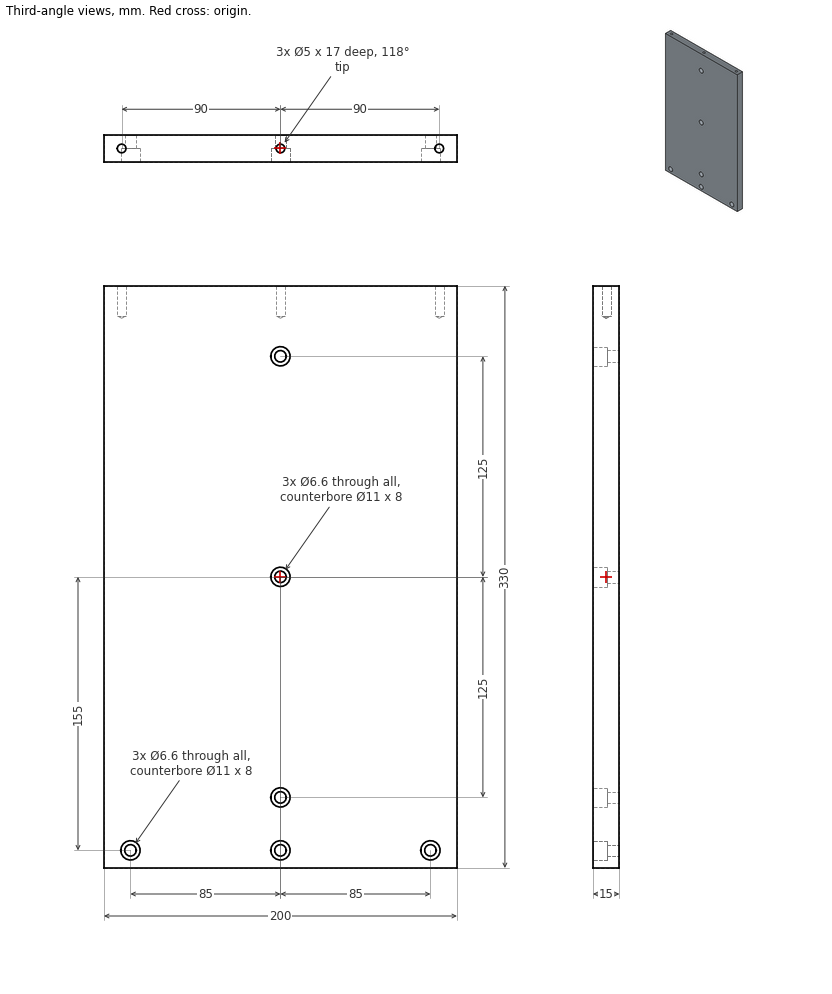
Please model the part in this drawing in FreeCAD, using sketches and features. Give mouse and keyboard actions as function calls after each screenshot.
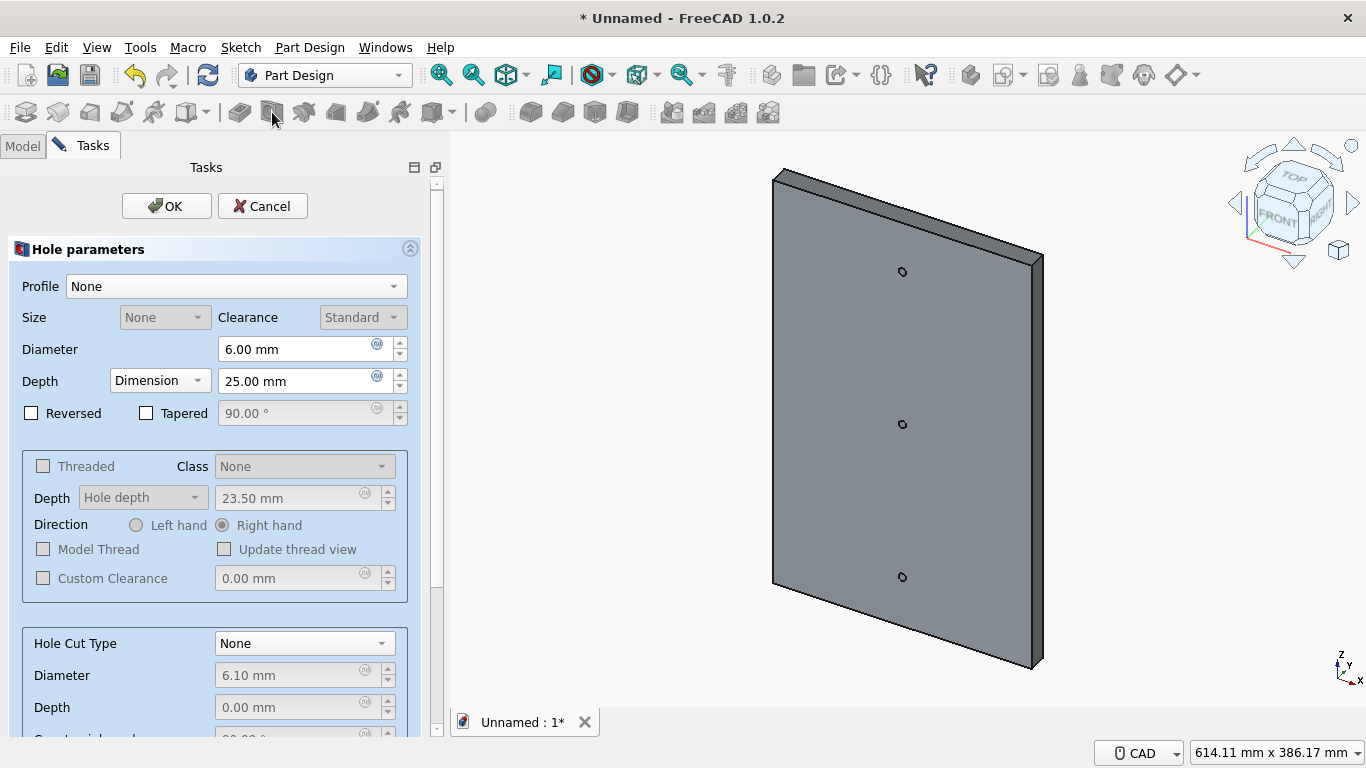
triple_click(305, 349)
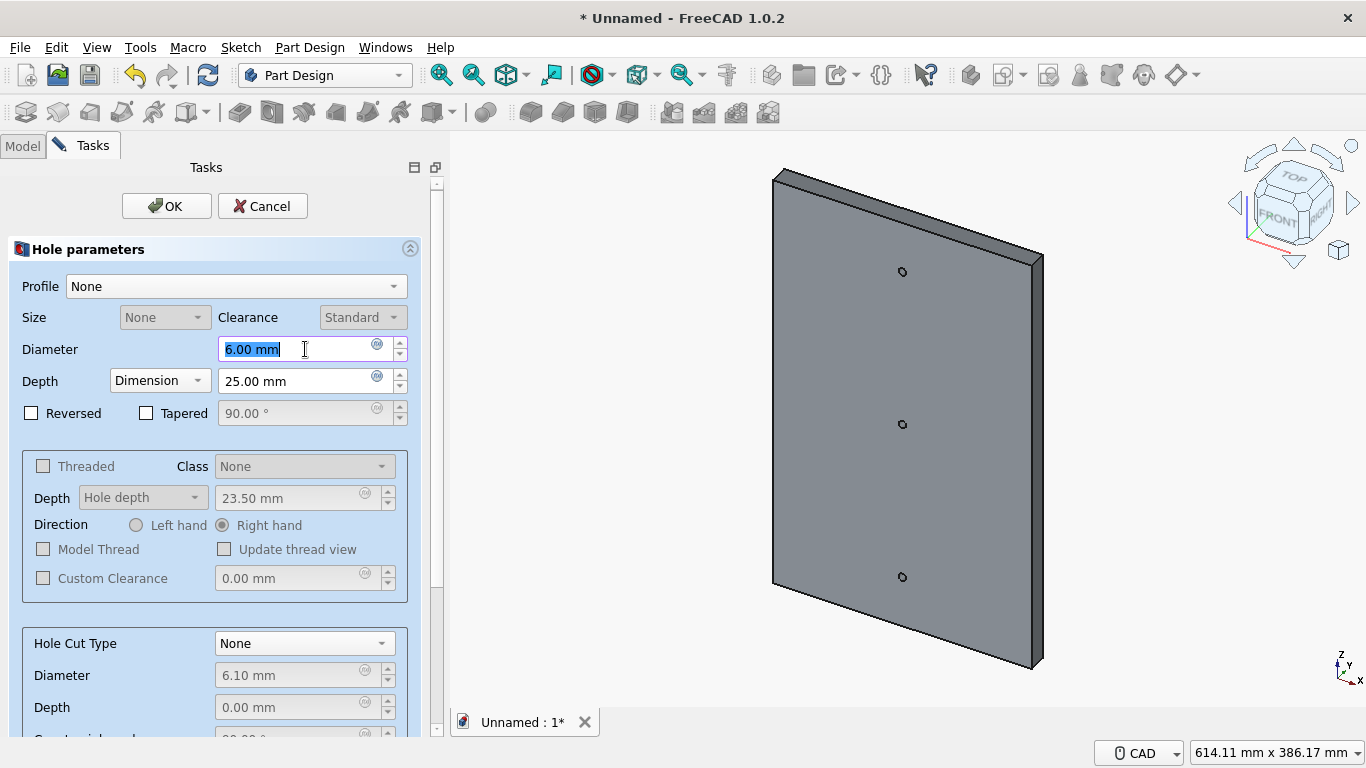
text(6.6)
key(Tab)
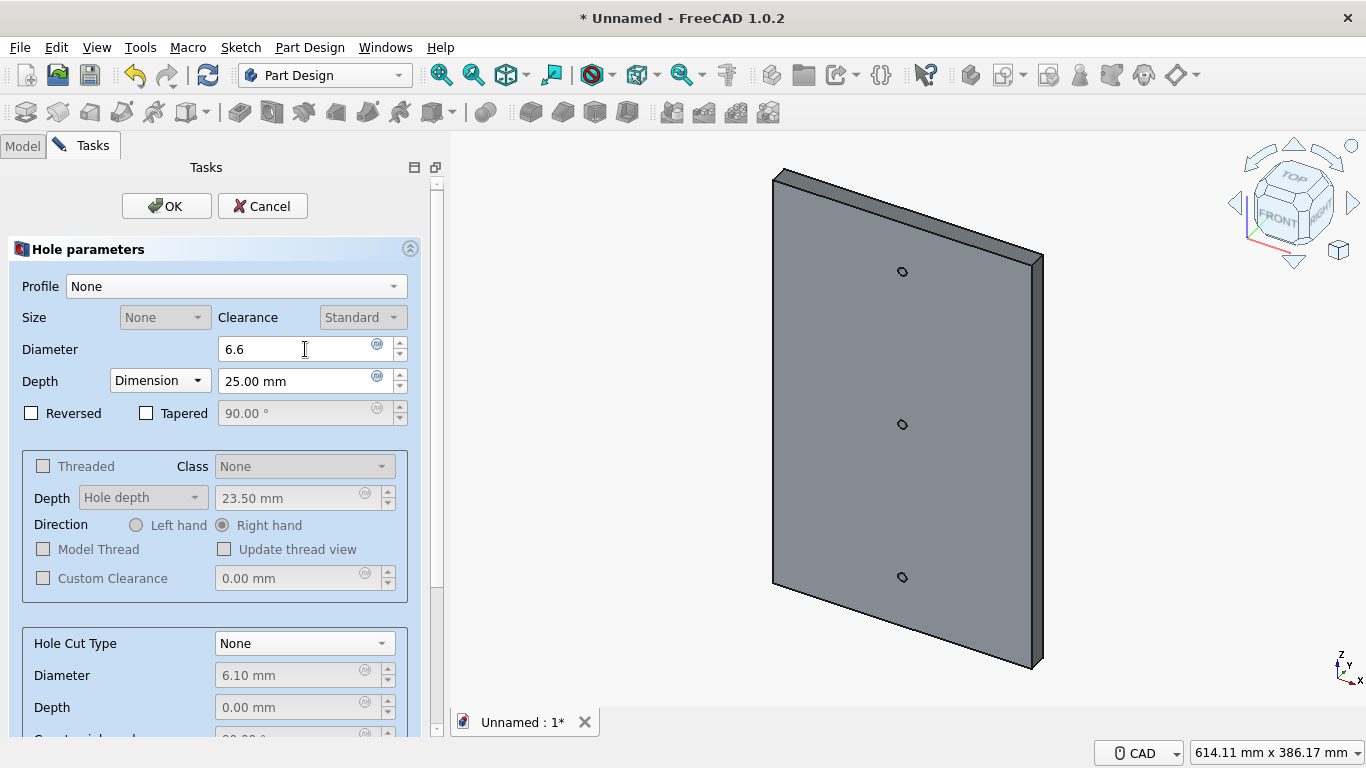
click(161, 380)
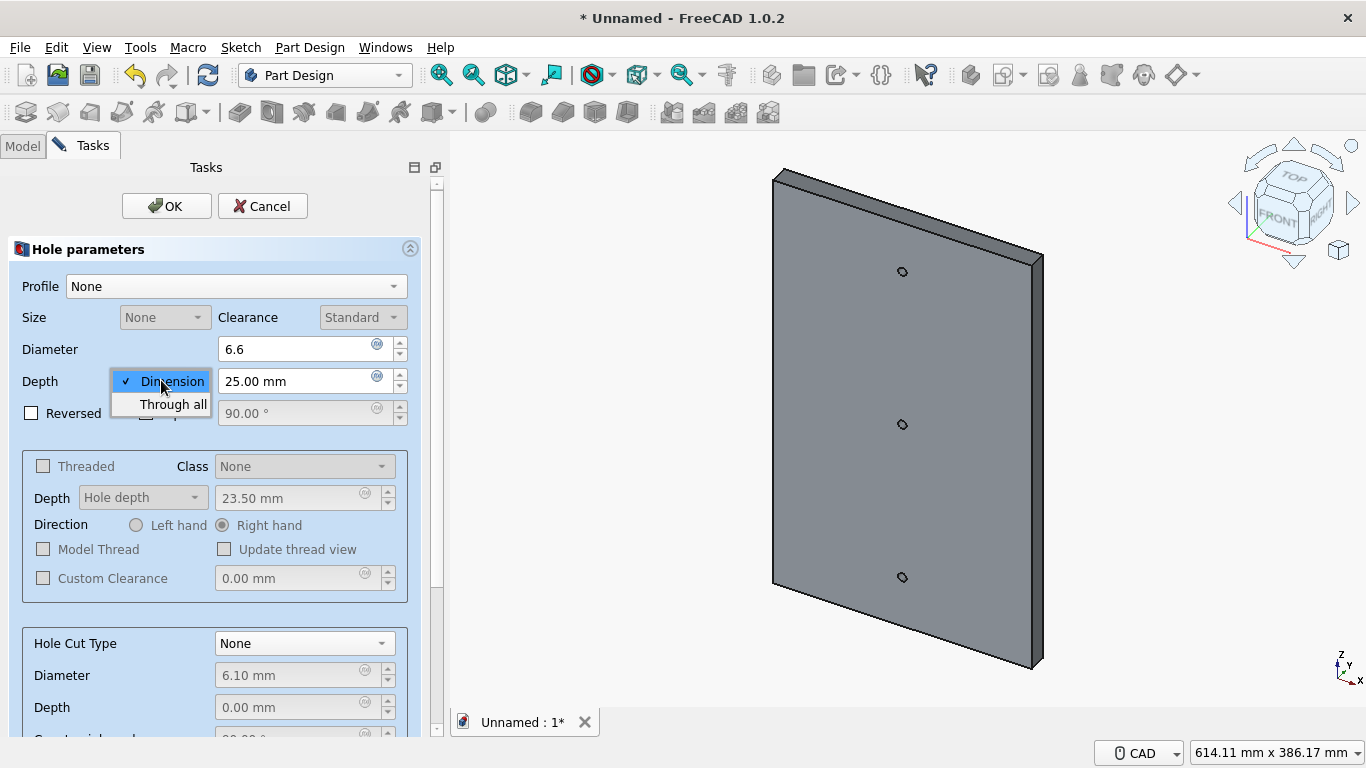
click(160, 404)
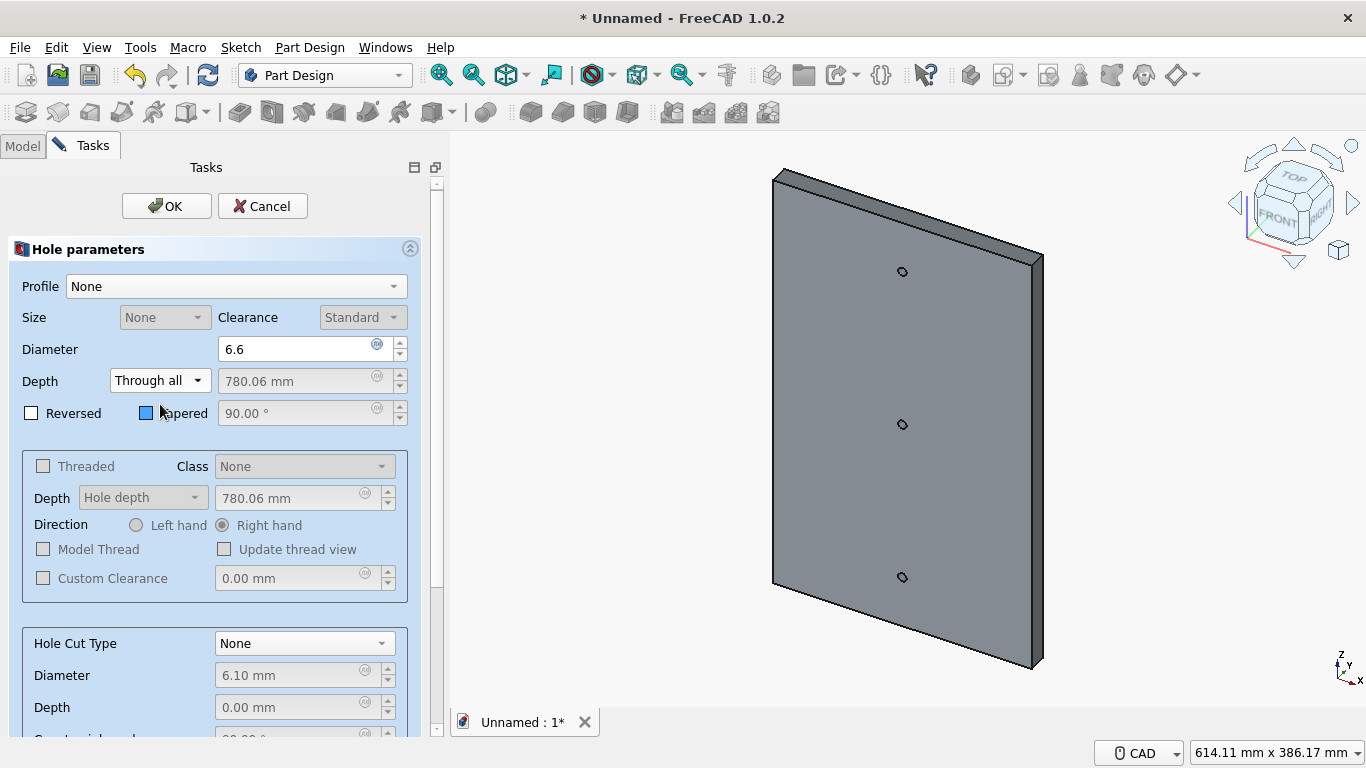
click(306, 644)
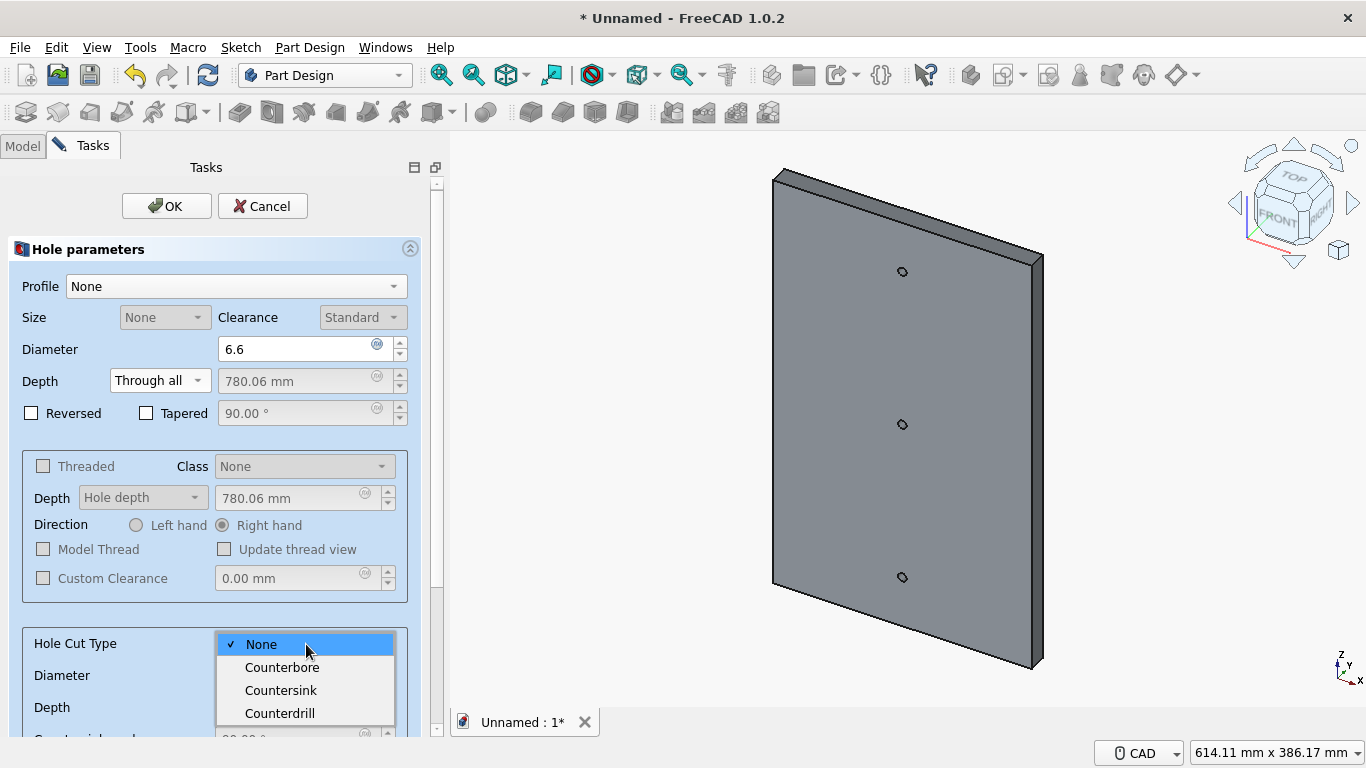
click(304, 668)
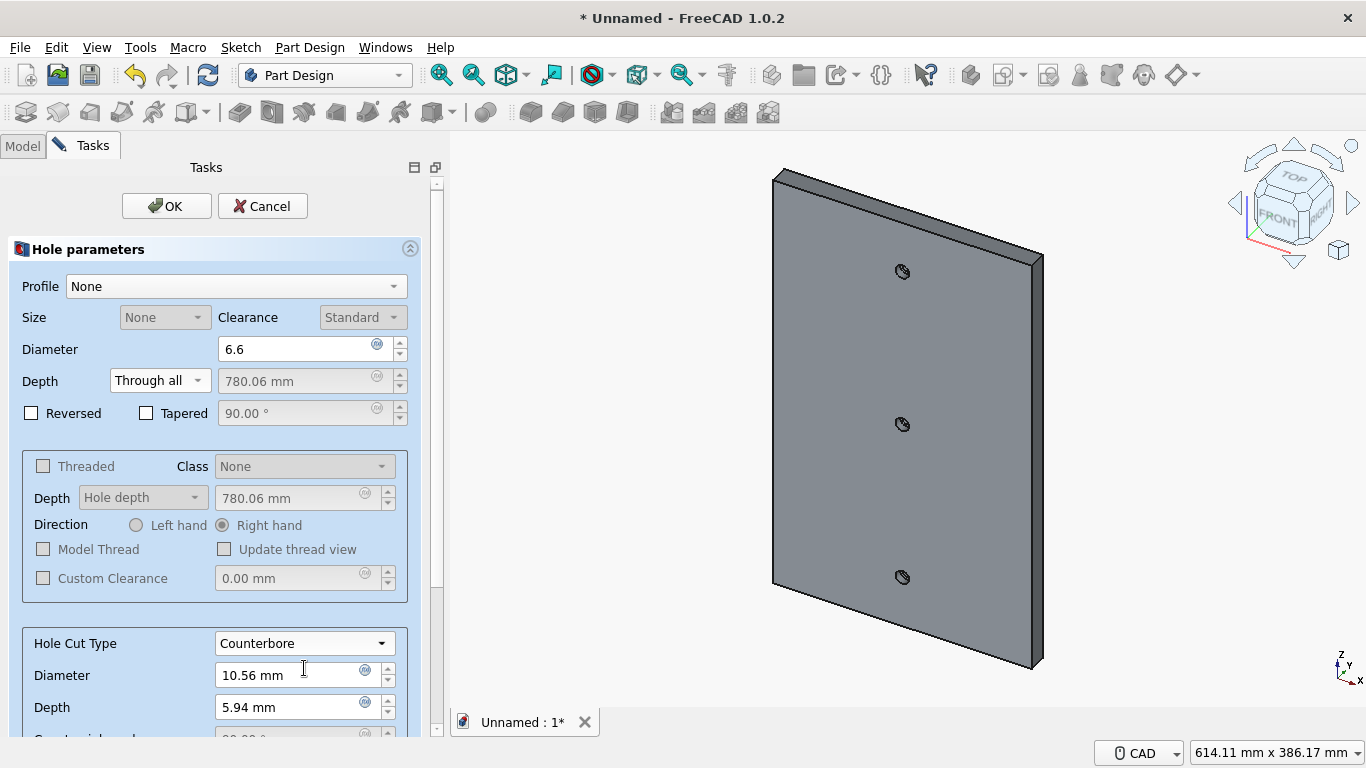
triple_click(298, 675)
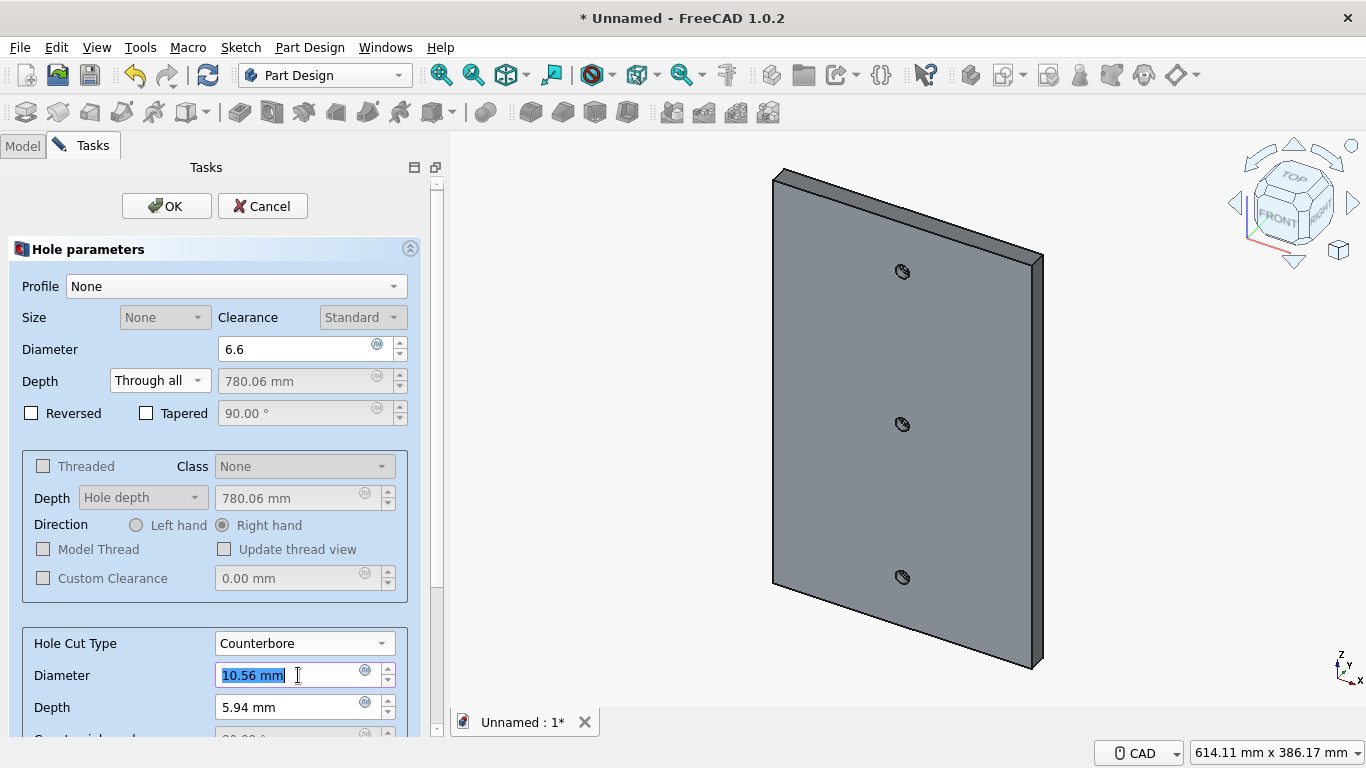
text(11)
key(Tab)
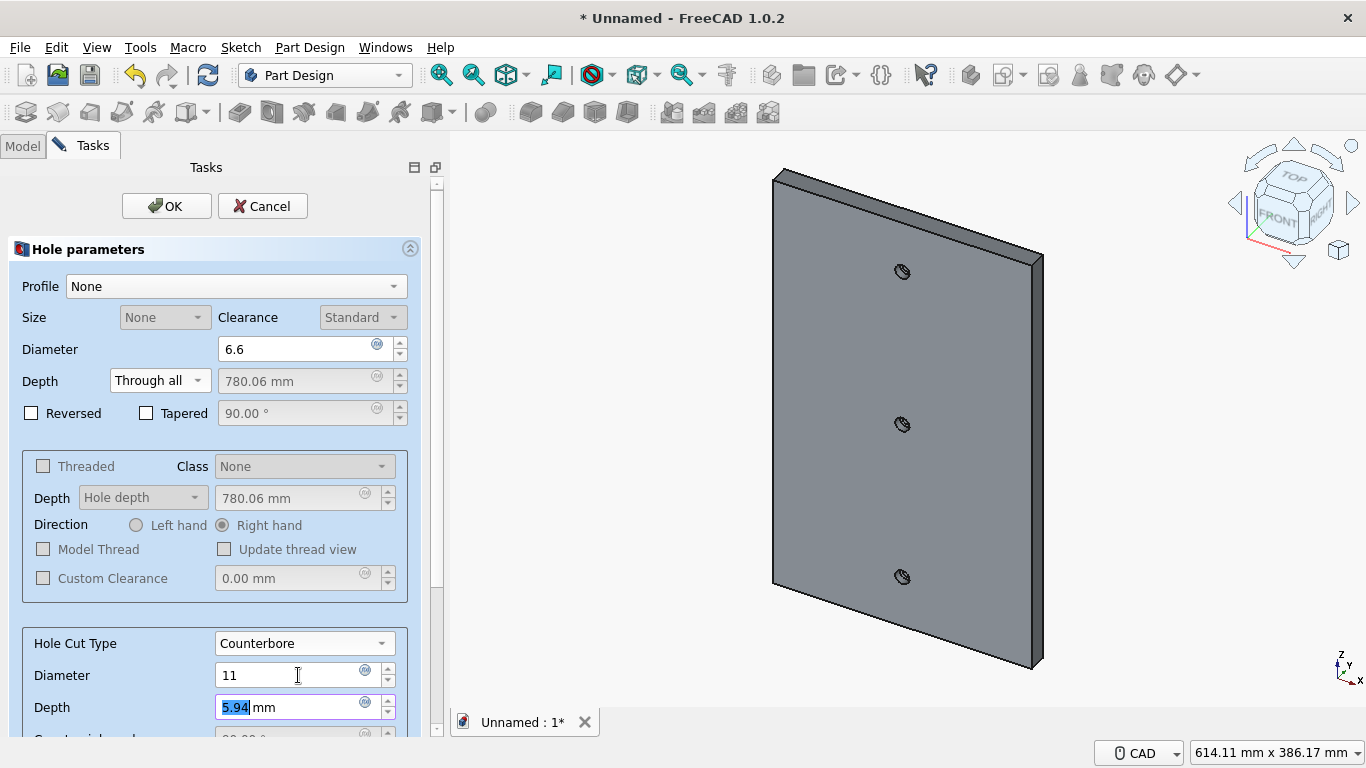
text(8)
key(Tab)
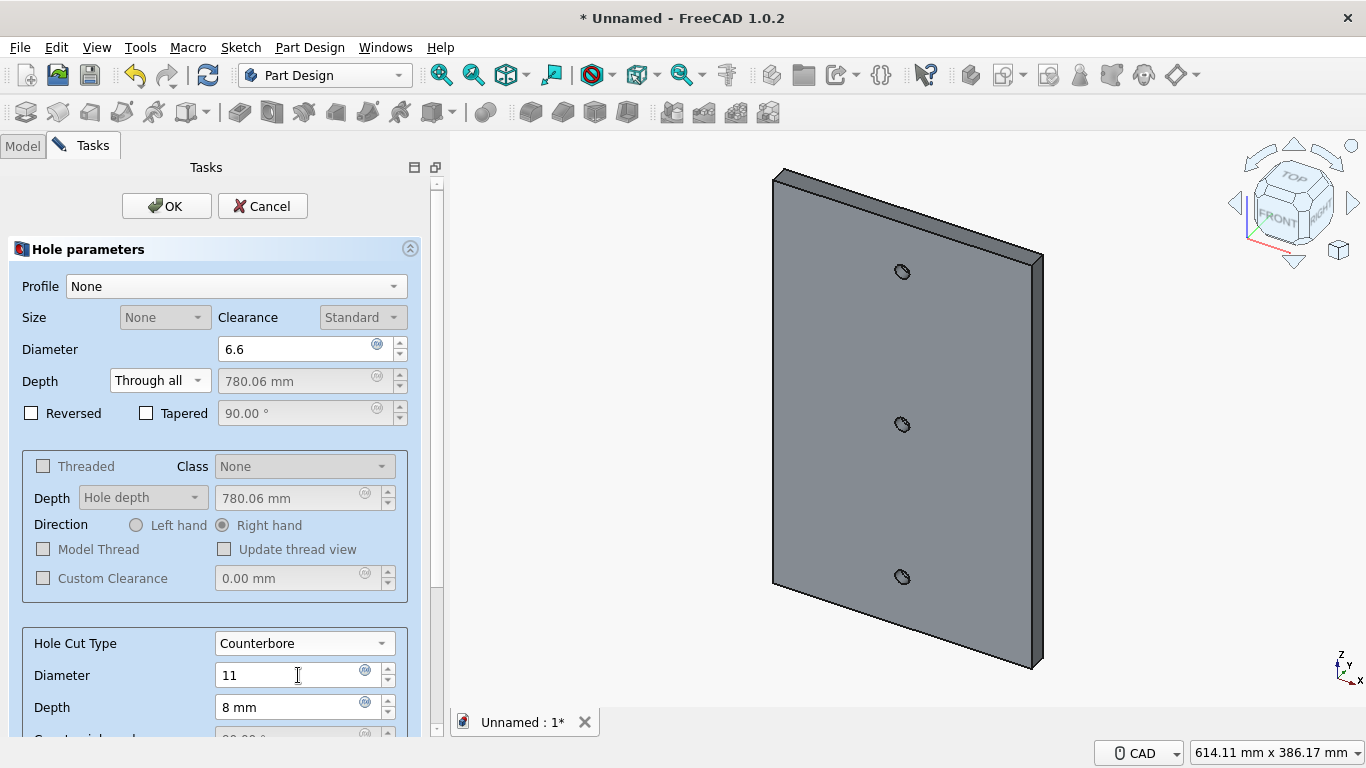
click(167, 206)